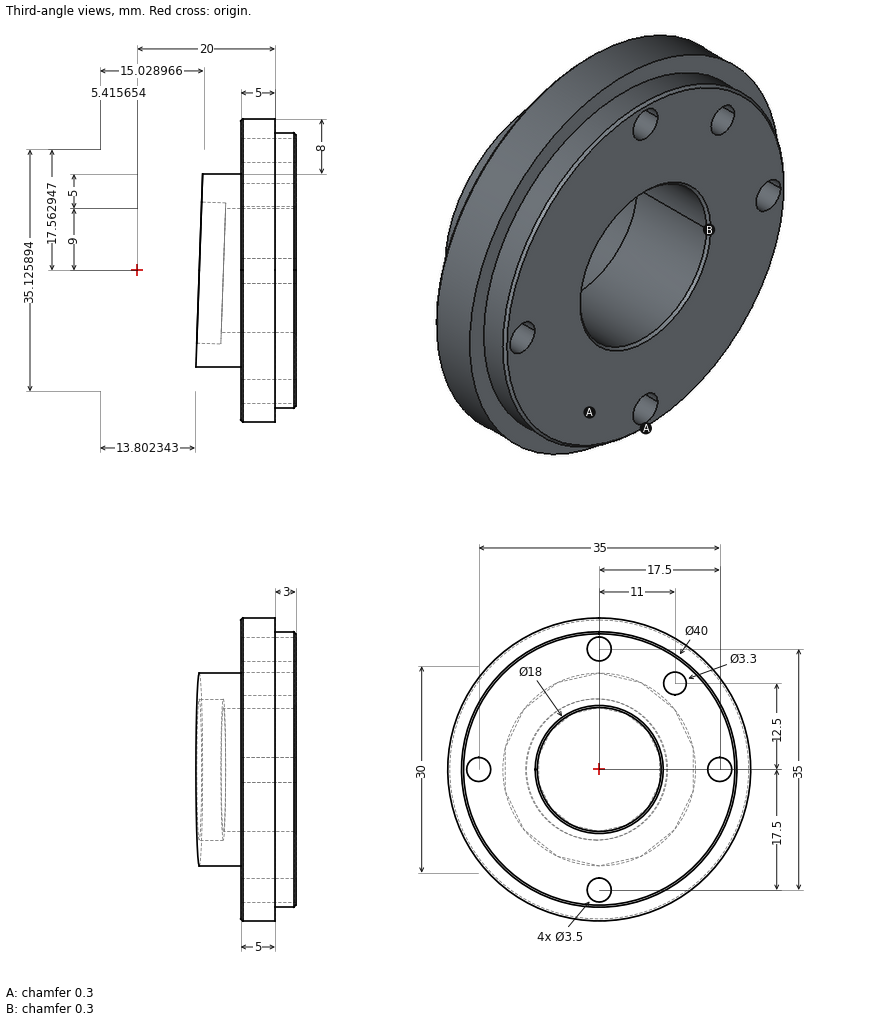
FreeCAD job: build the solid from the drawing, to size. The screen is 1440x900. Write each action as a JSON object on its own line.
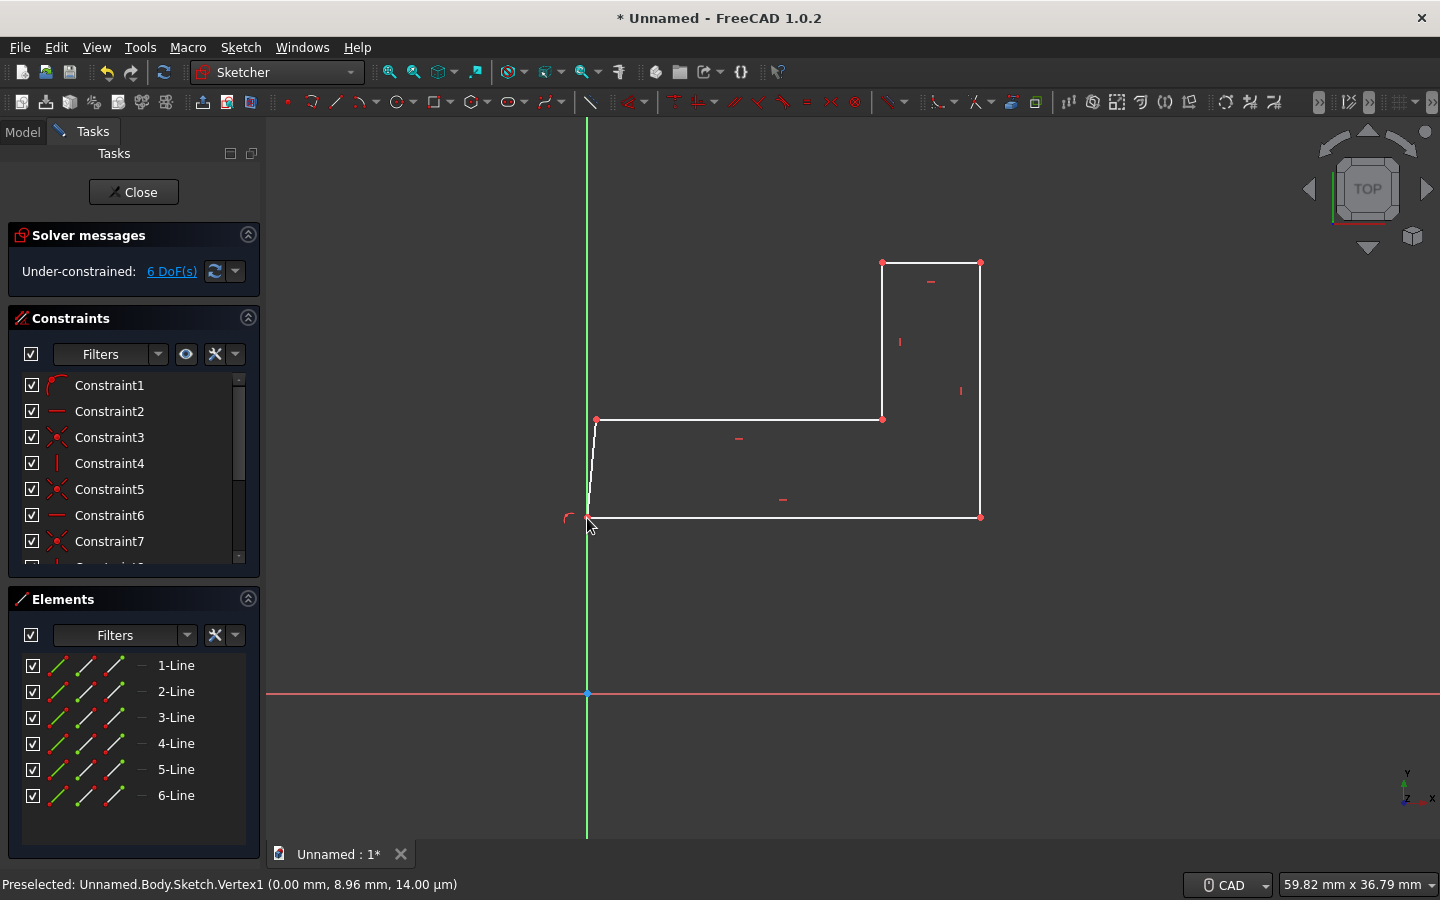
{"action": "left_click", "coordinate": [590, 489]}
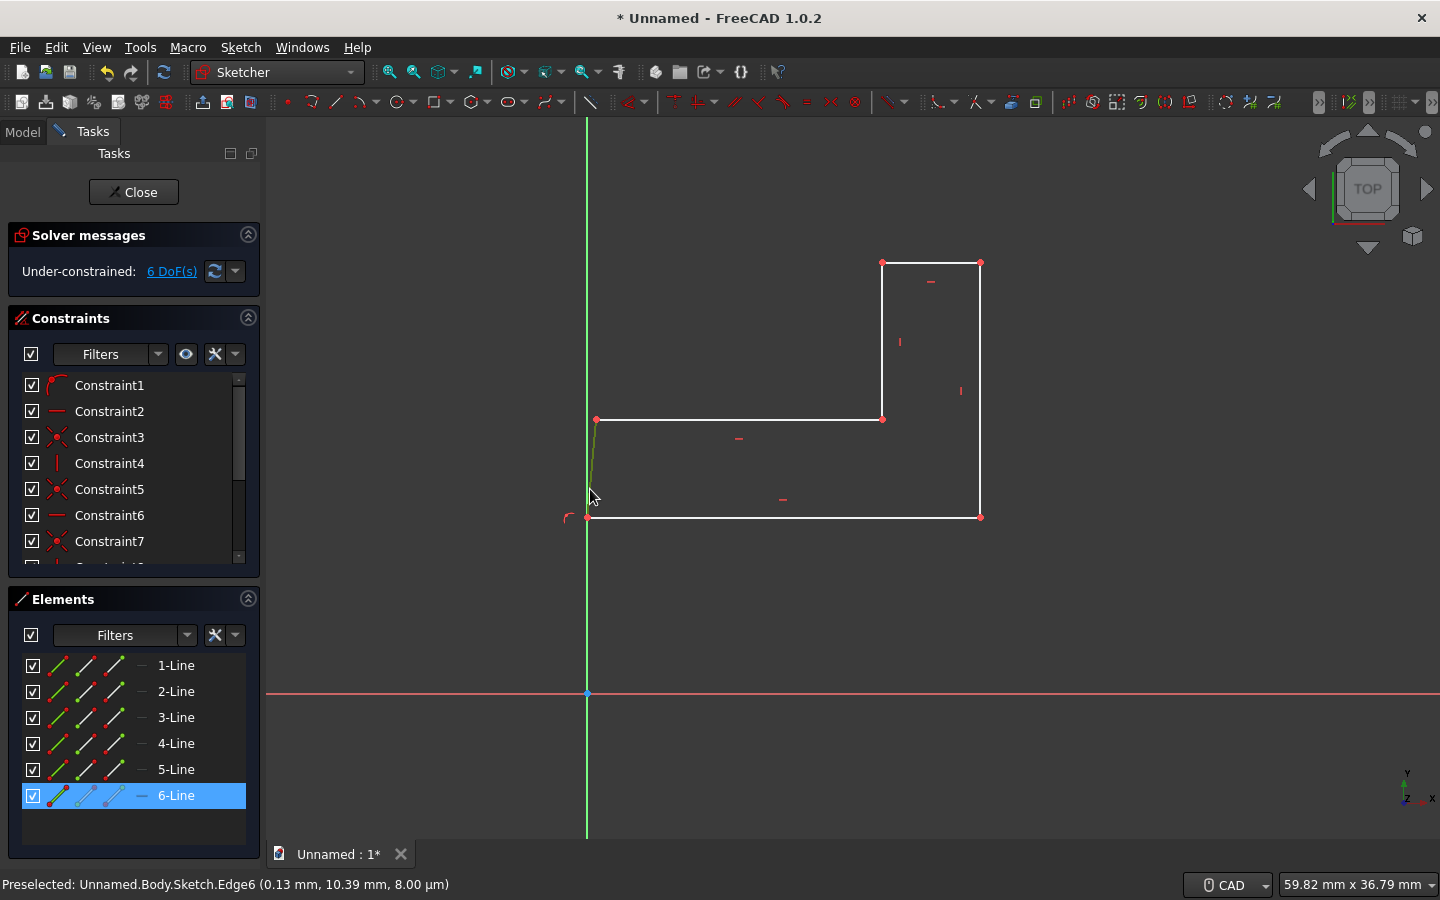
{"action": "key", "text": "v"}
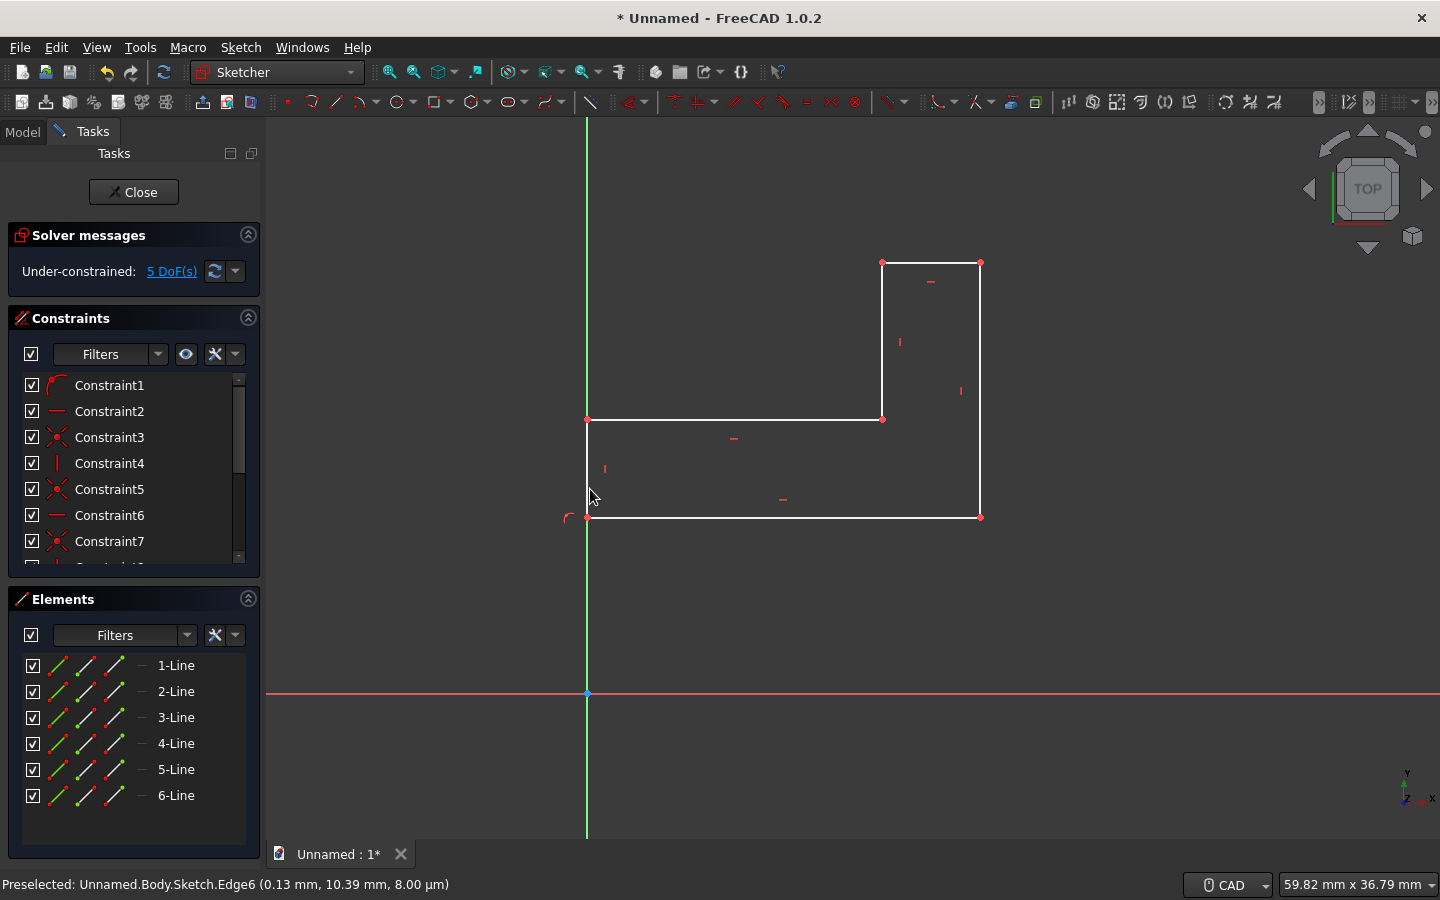
{"action": "left_click", "coordinate": [951, 263]}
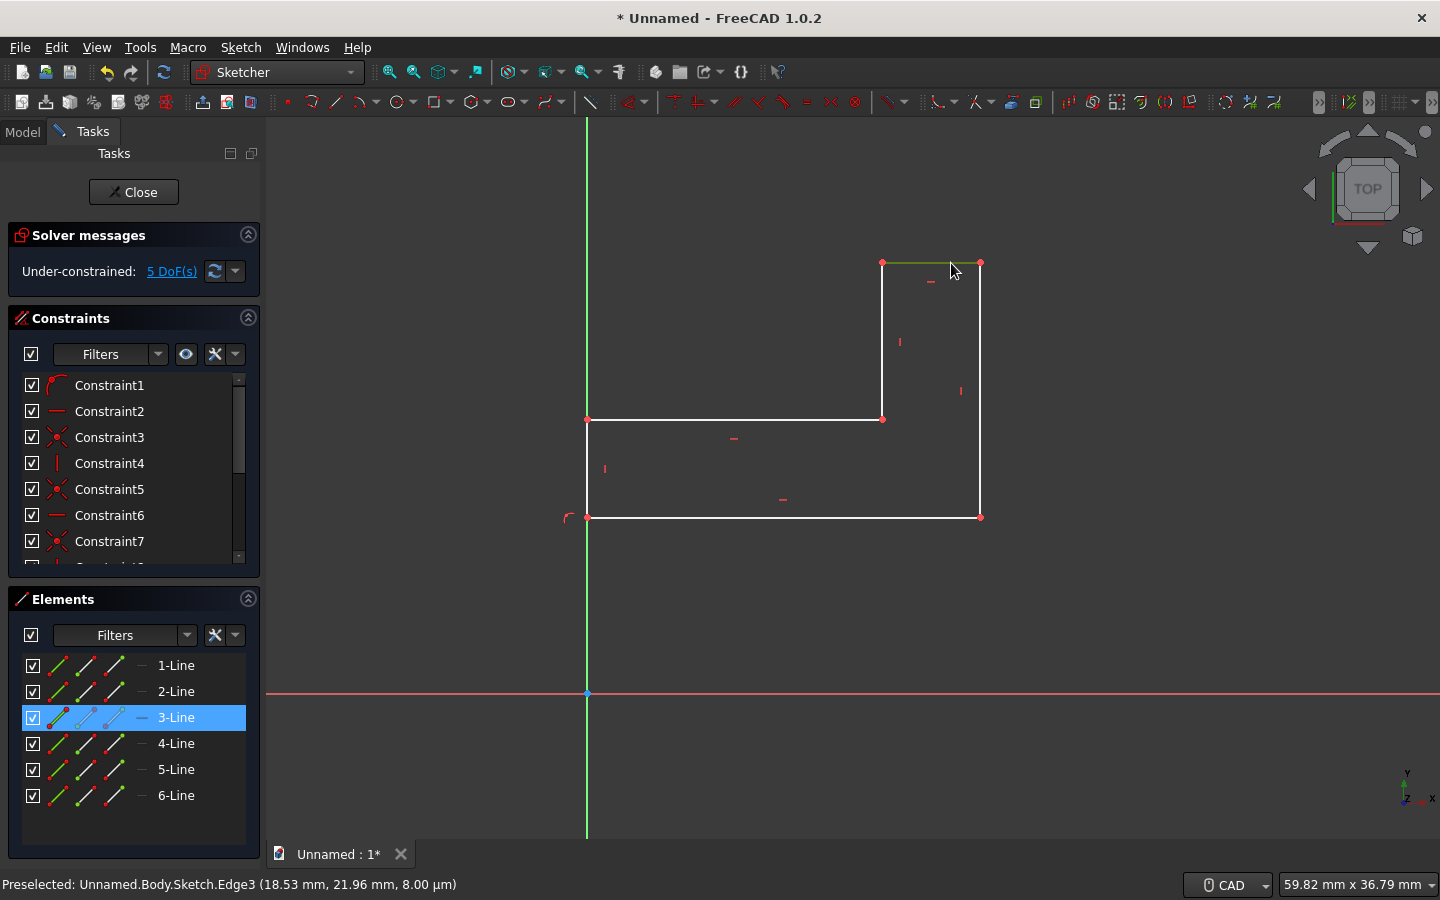
{"action": "left_click", "coordinate": [646, 102]}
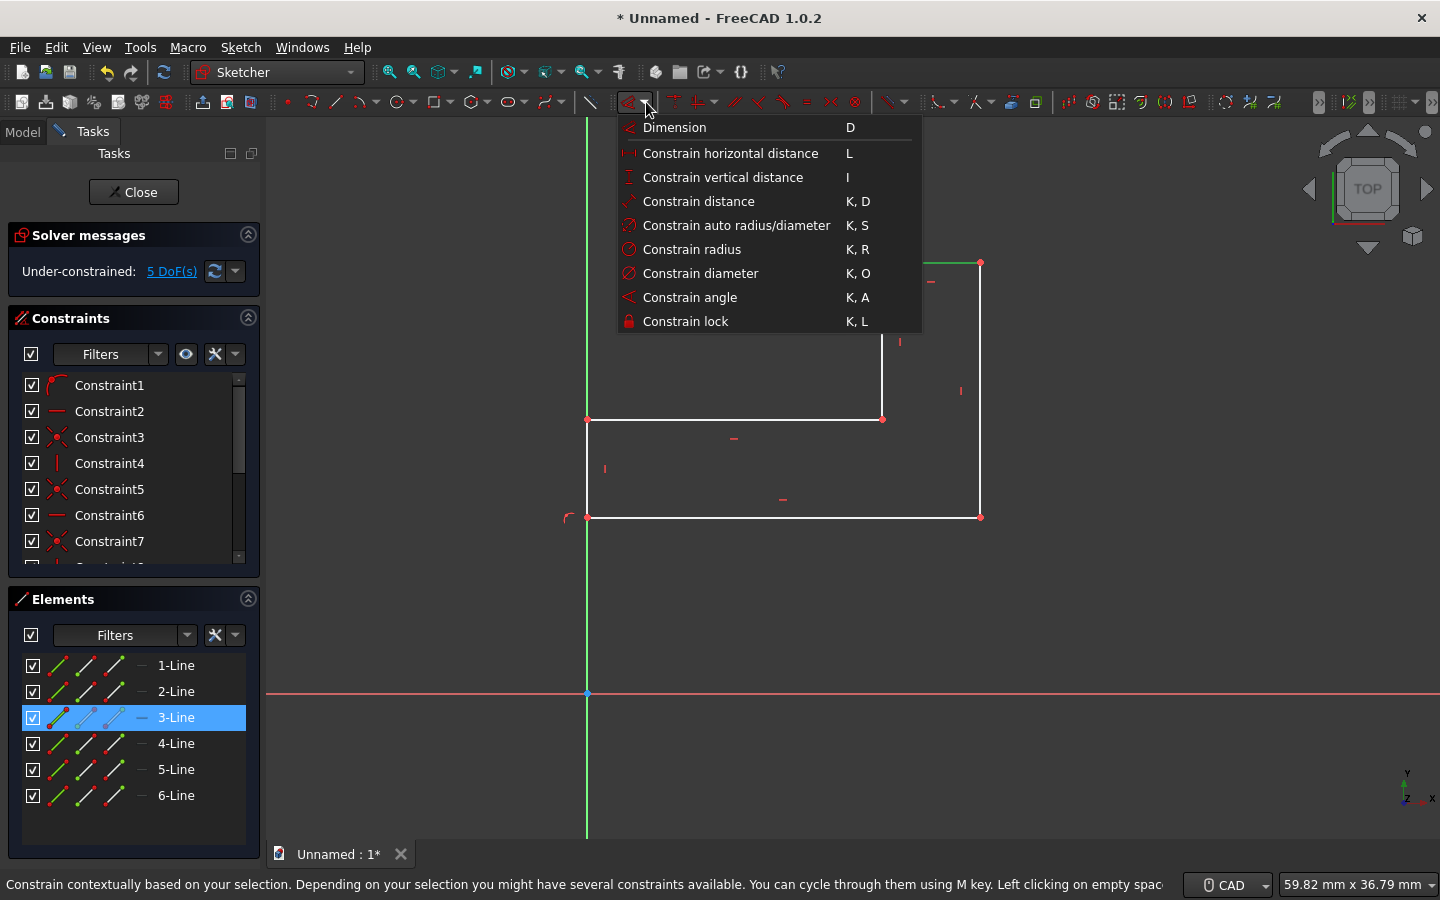
{"action": "left_click", "coordinate": [770, 153]}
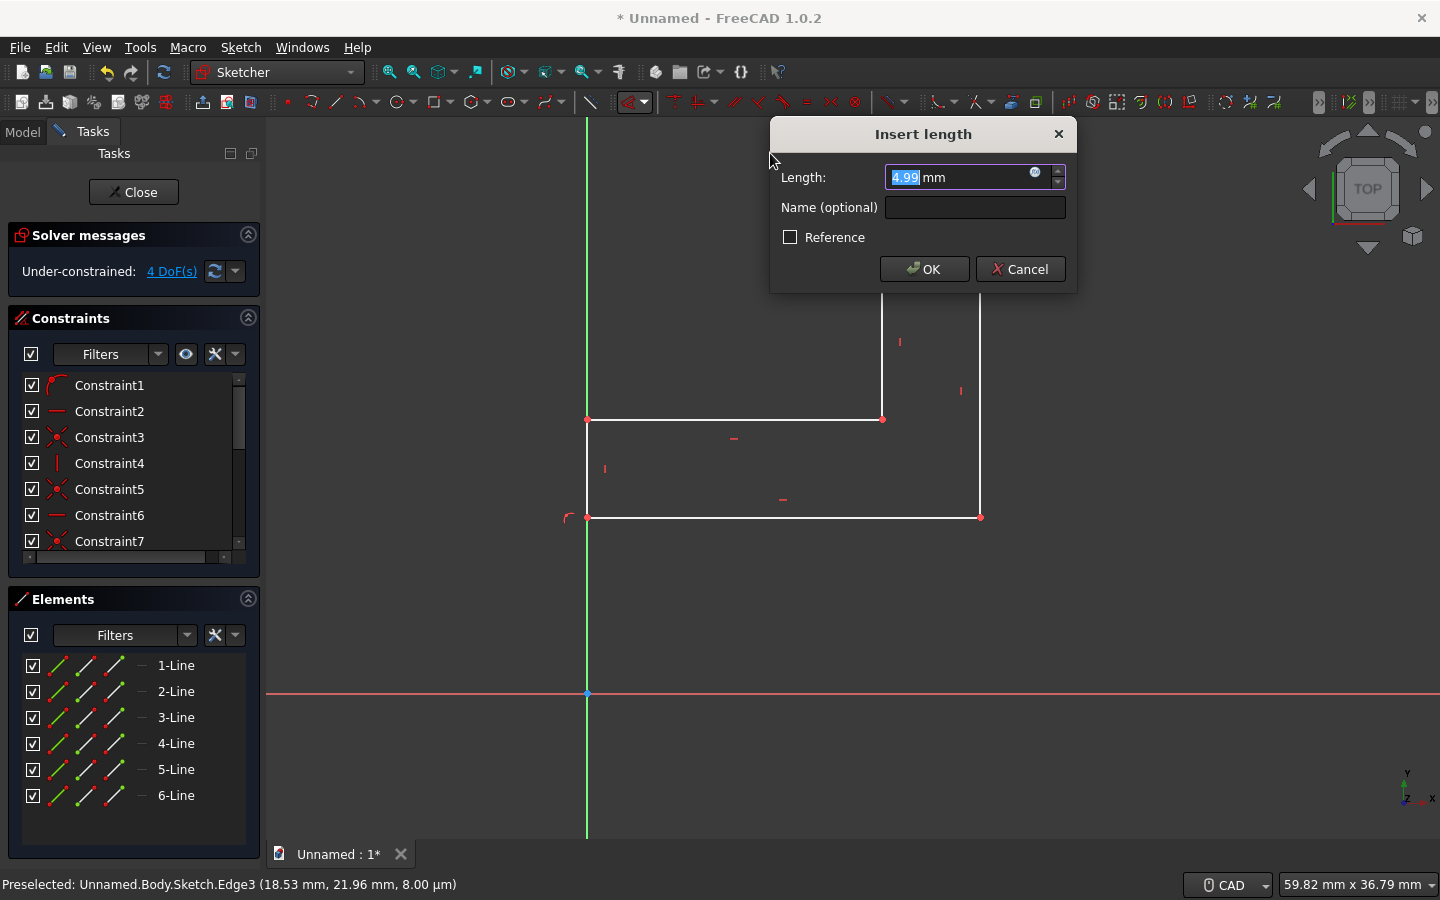
{"action": "type", "text": "5"}
{"action": "key", "text": "Return"}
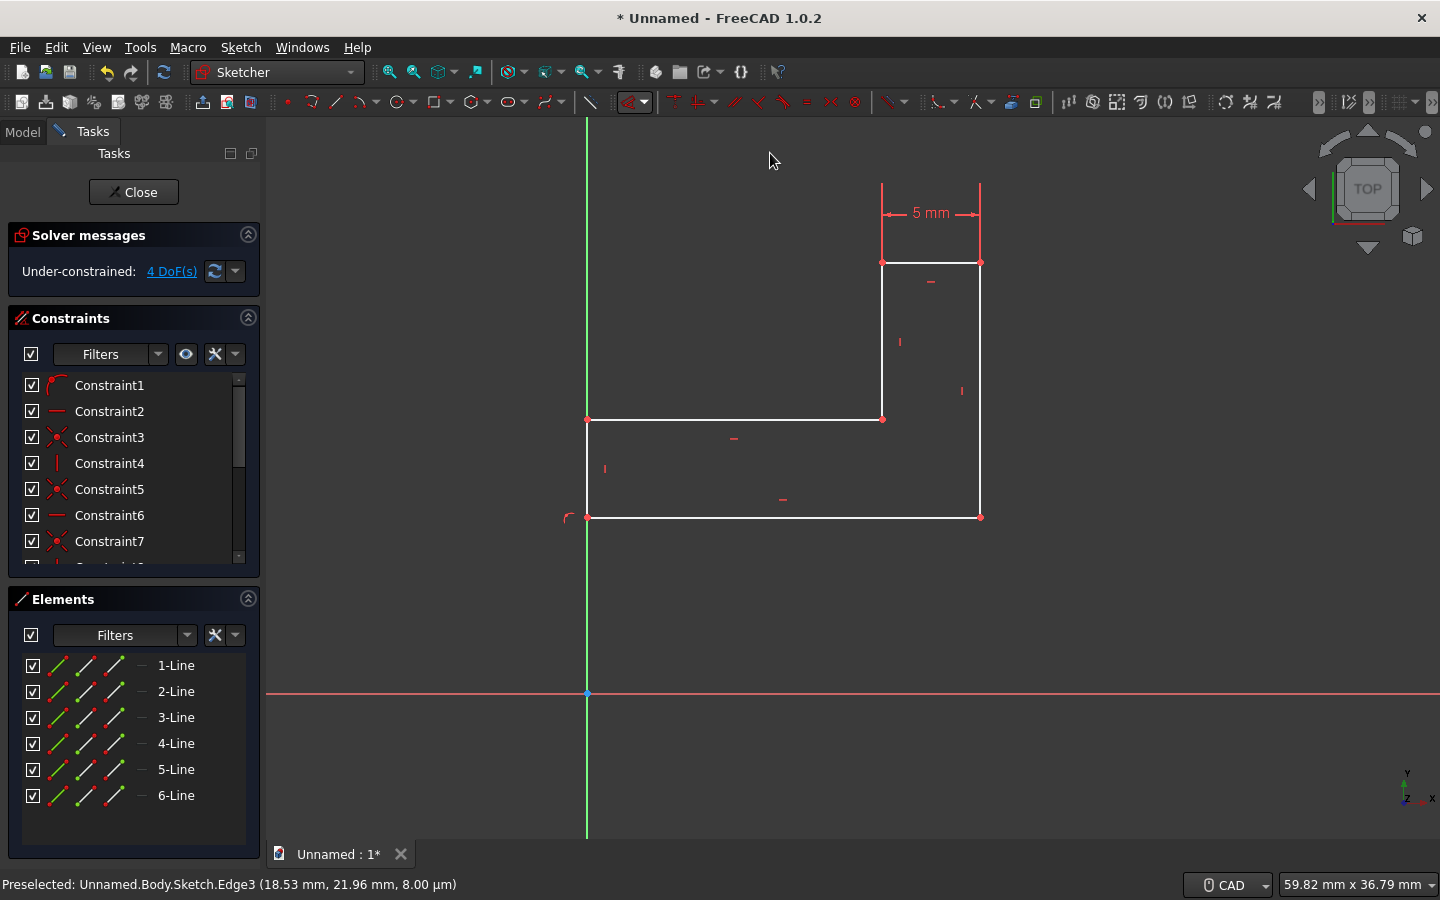
{"action": "left_click", "coordinate": [882, 310]}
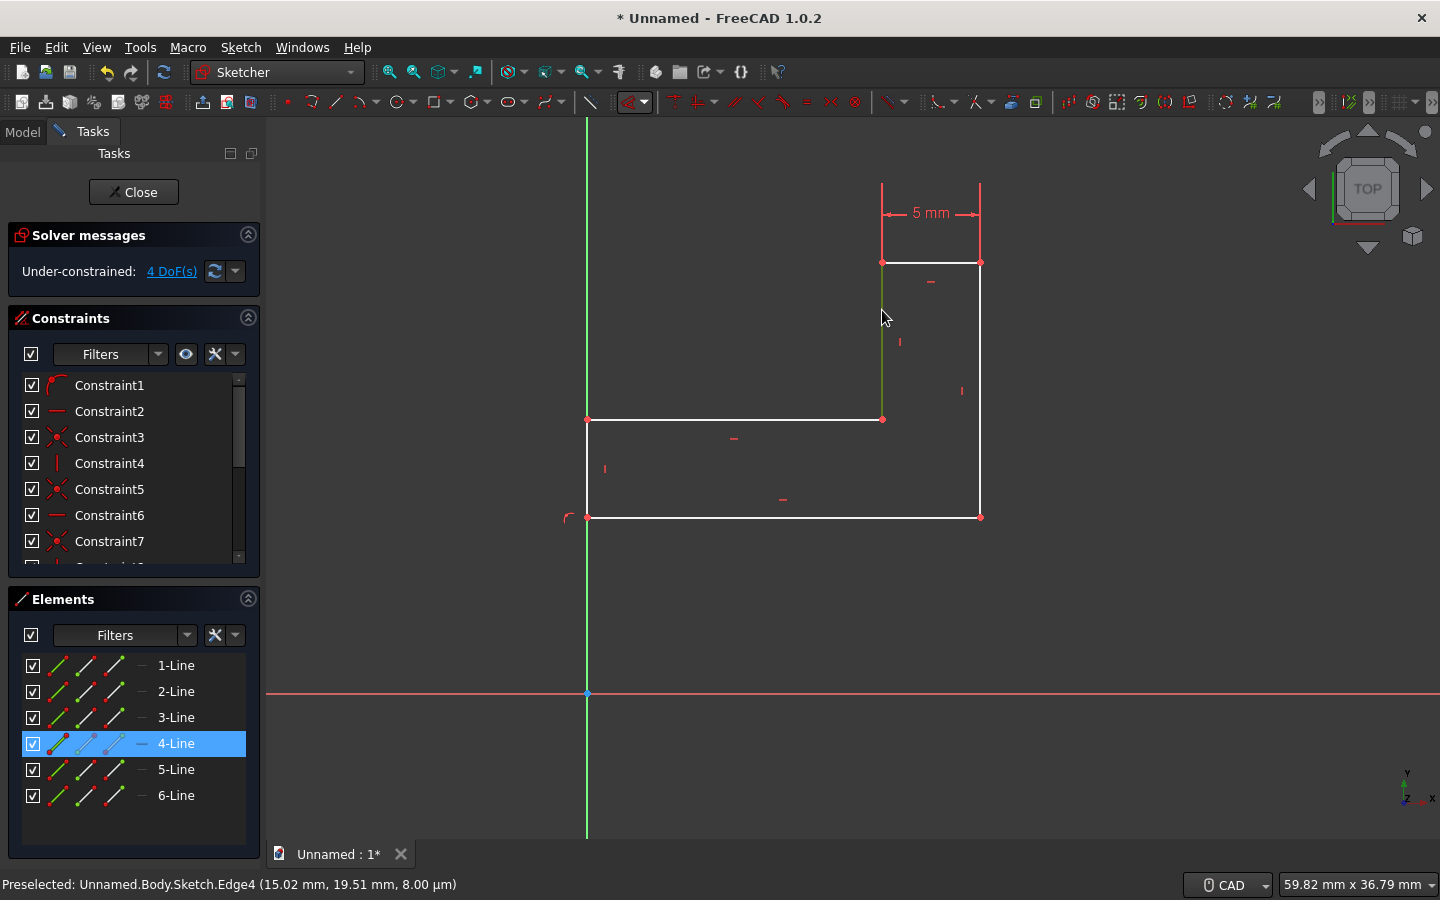
{"action": "key", "text": "i"}